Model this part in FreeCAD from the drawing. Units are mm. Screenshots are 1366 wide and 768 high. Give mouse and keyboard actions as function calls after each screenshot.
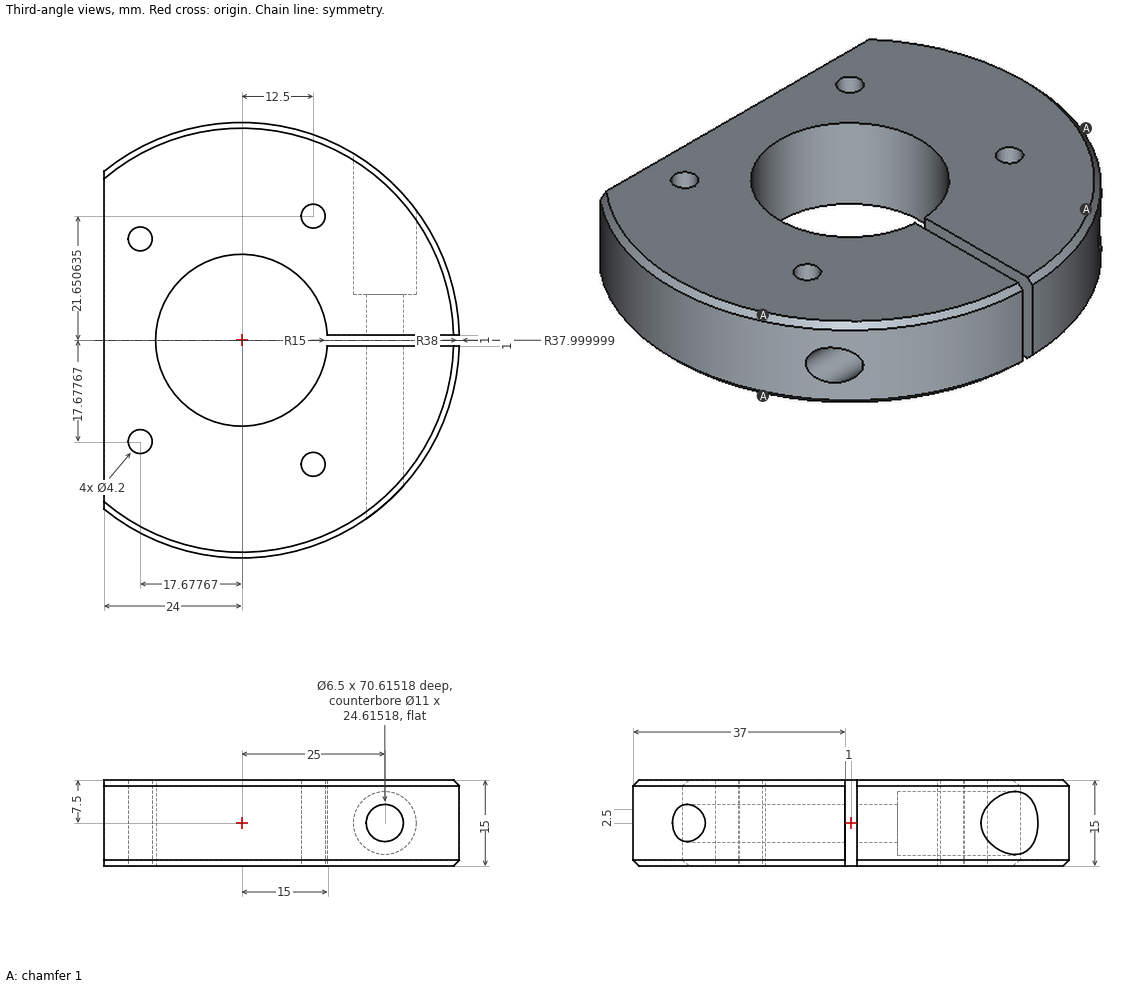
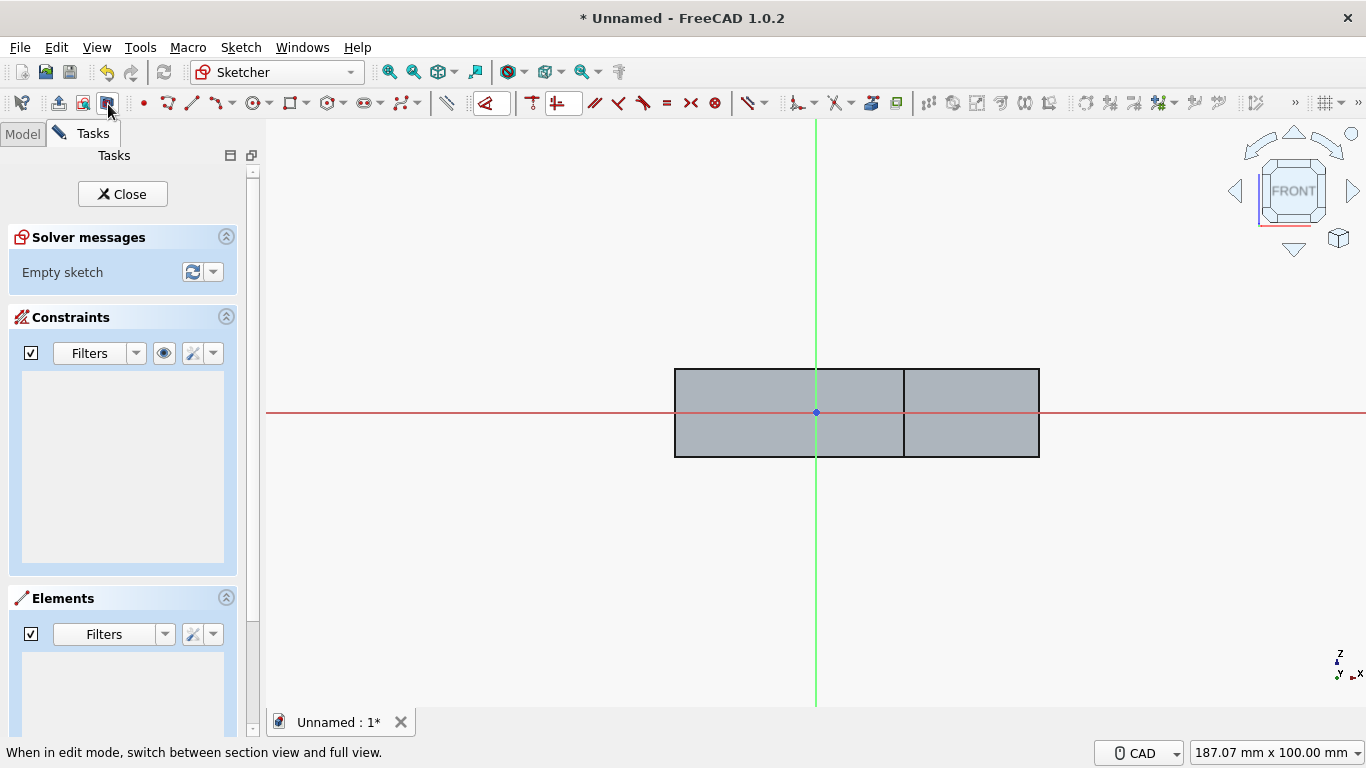
scroll(897, 413, up, 7)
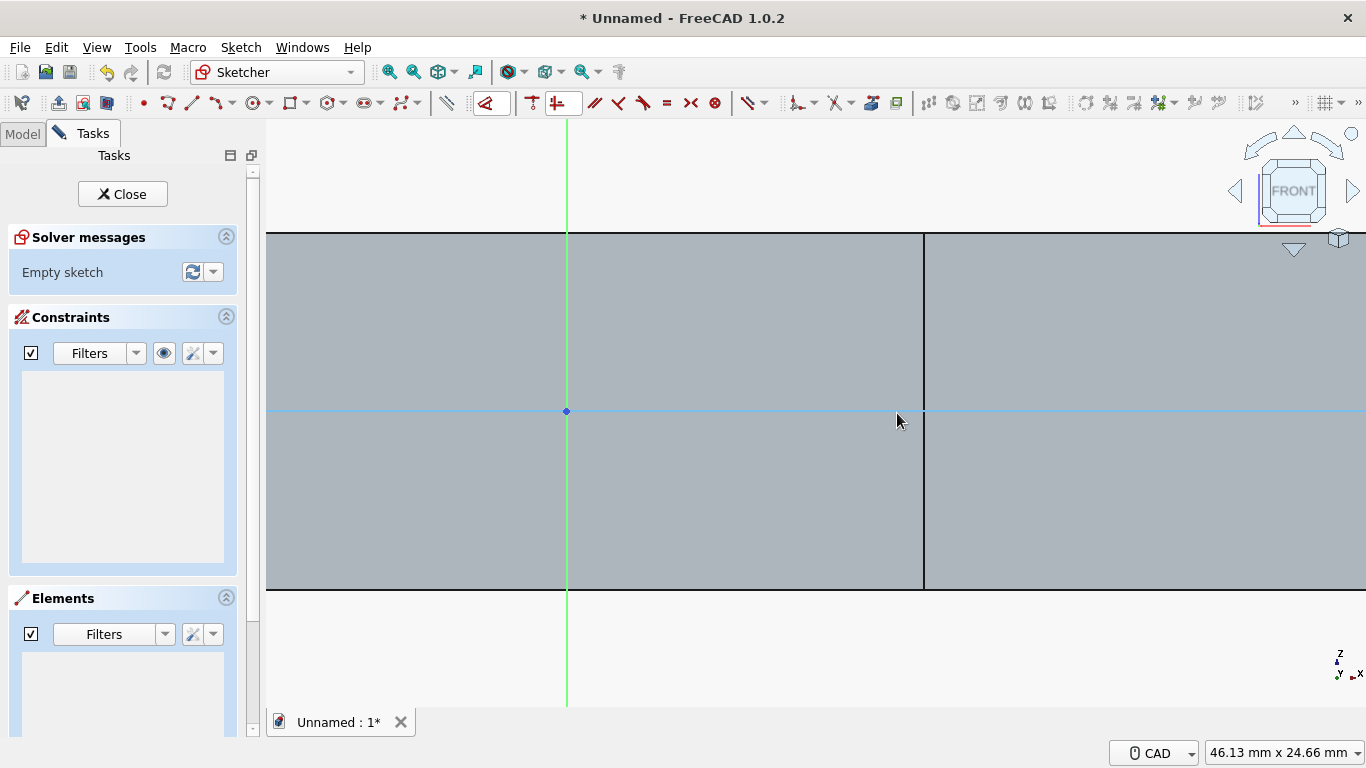
key(g)
key(r)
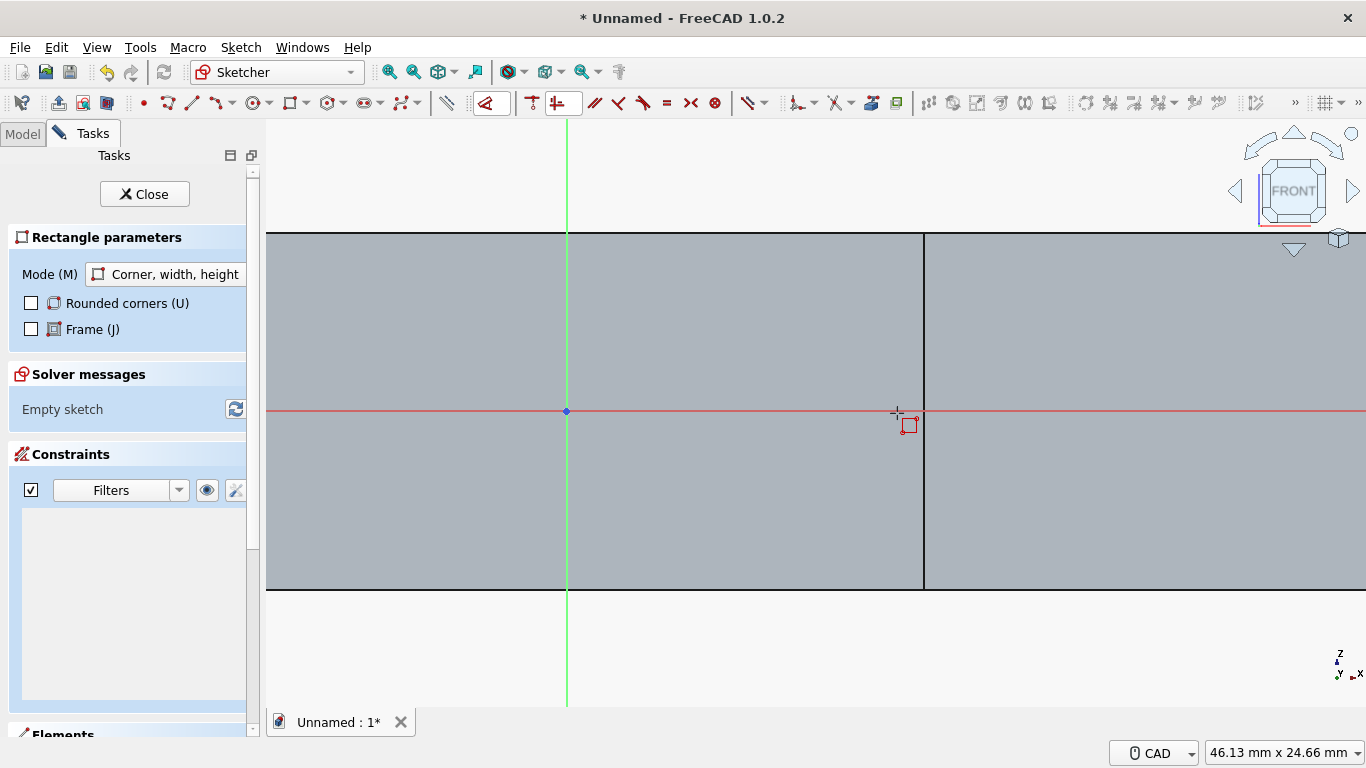
click(567, 233)
move(924, 590)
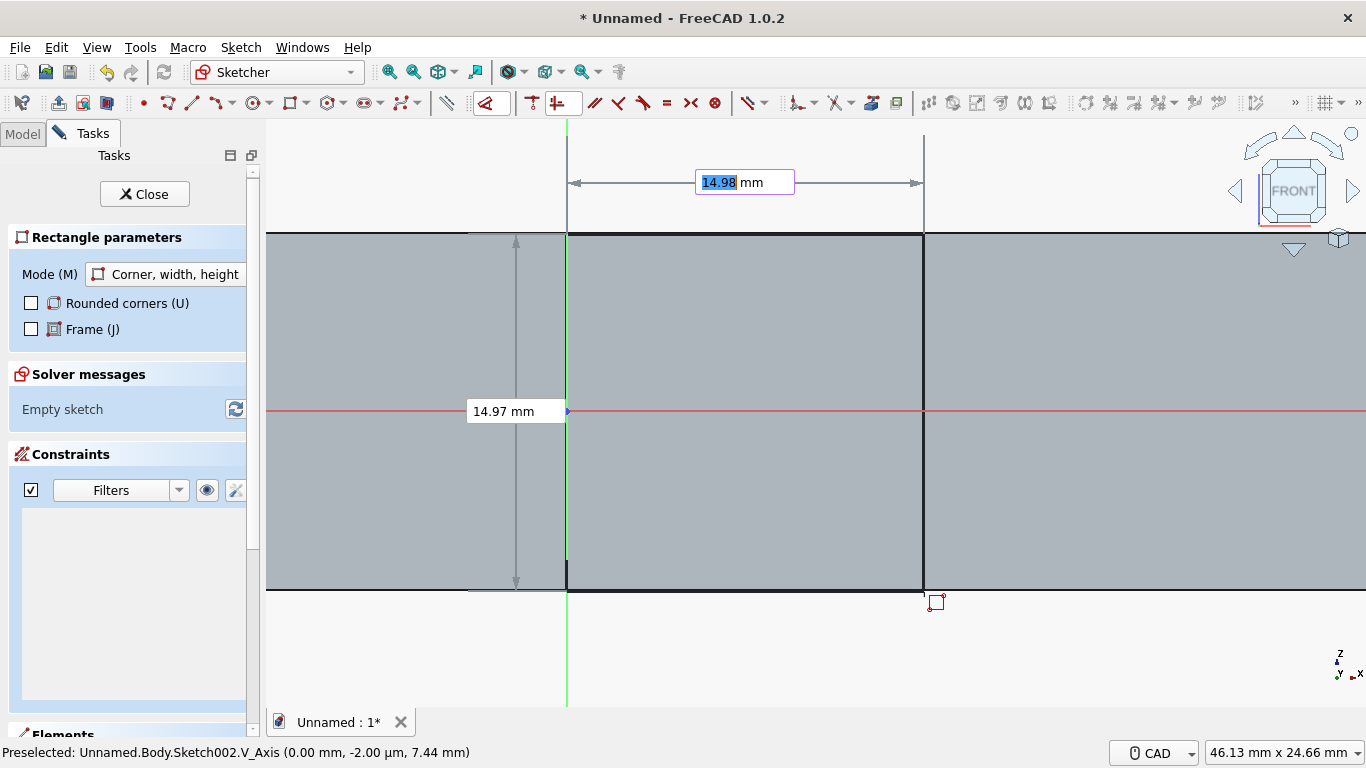
text(15)
key(Tab)
text(15)
key(Return)
key(Escape)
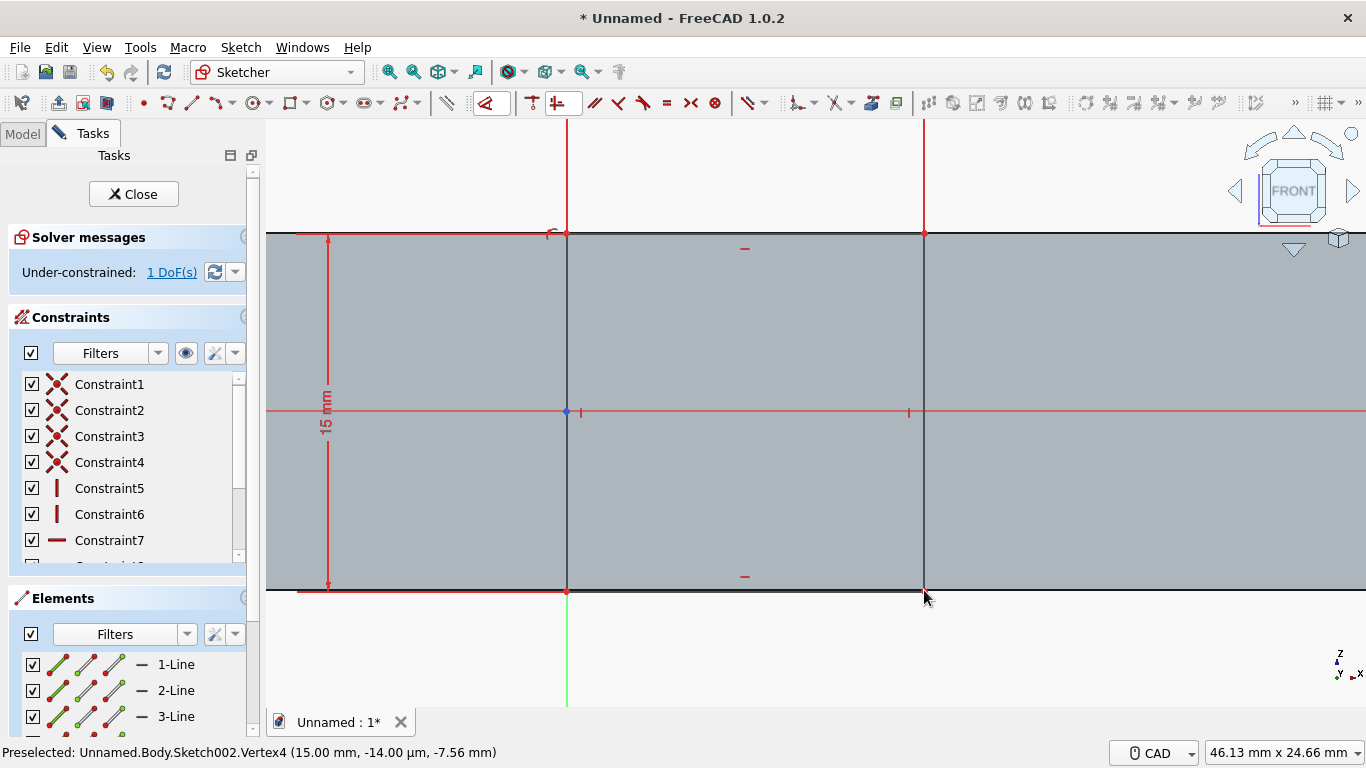
click(567, 234)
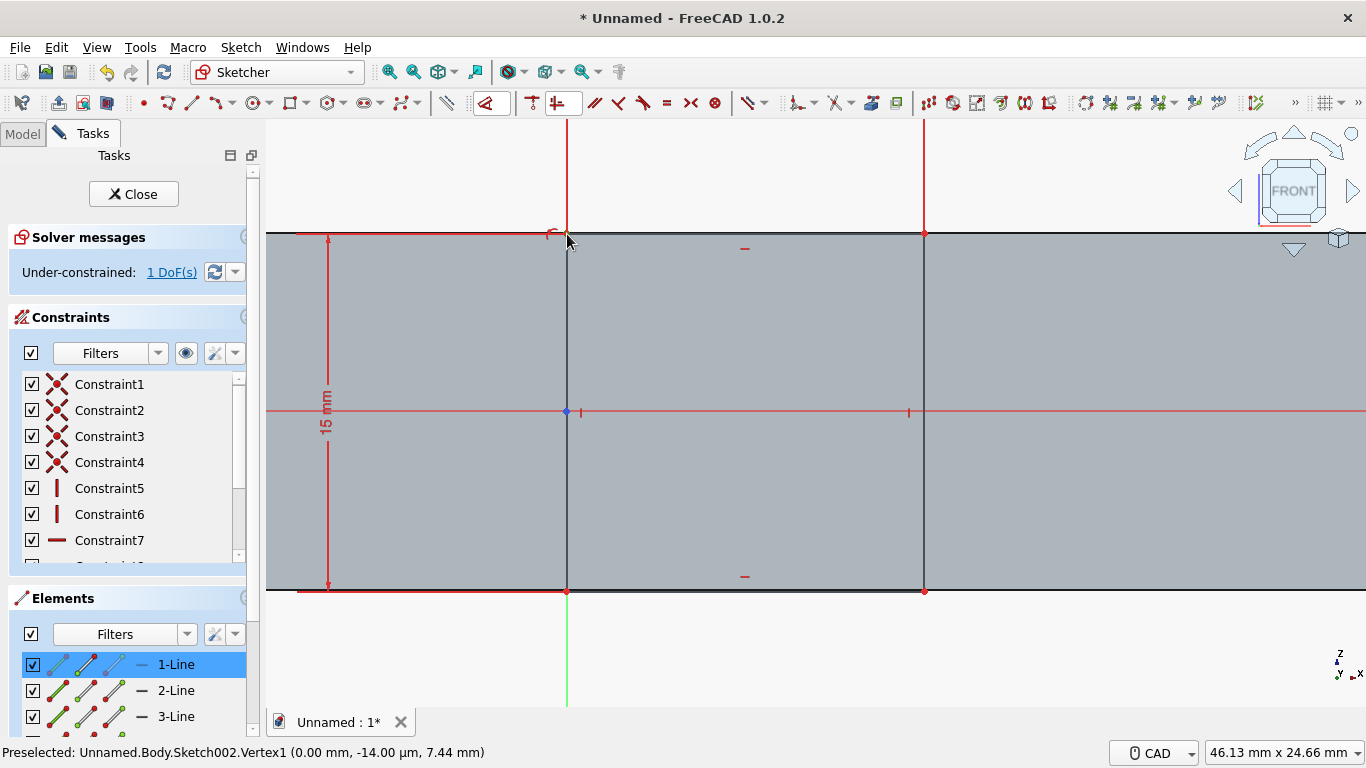
click(504, 104)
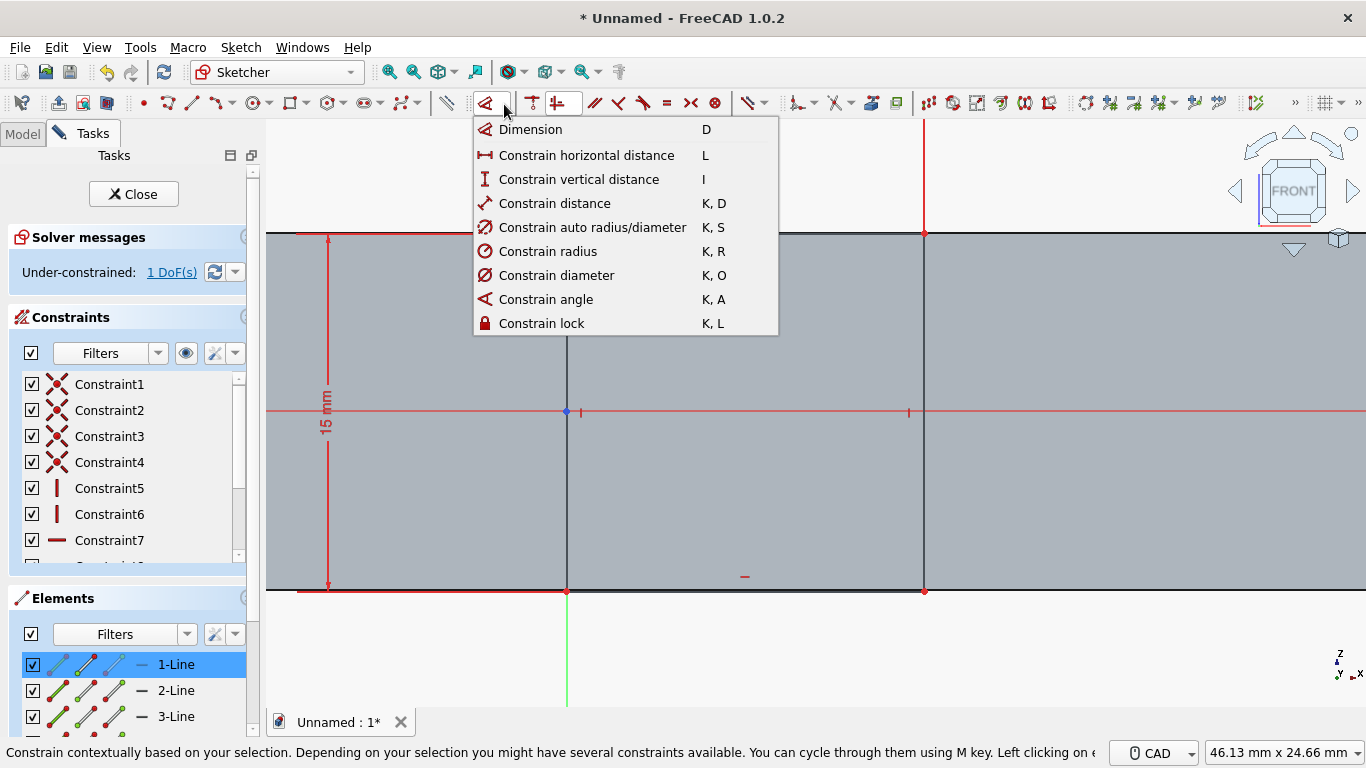
click(626, 179)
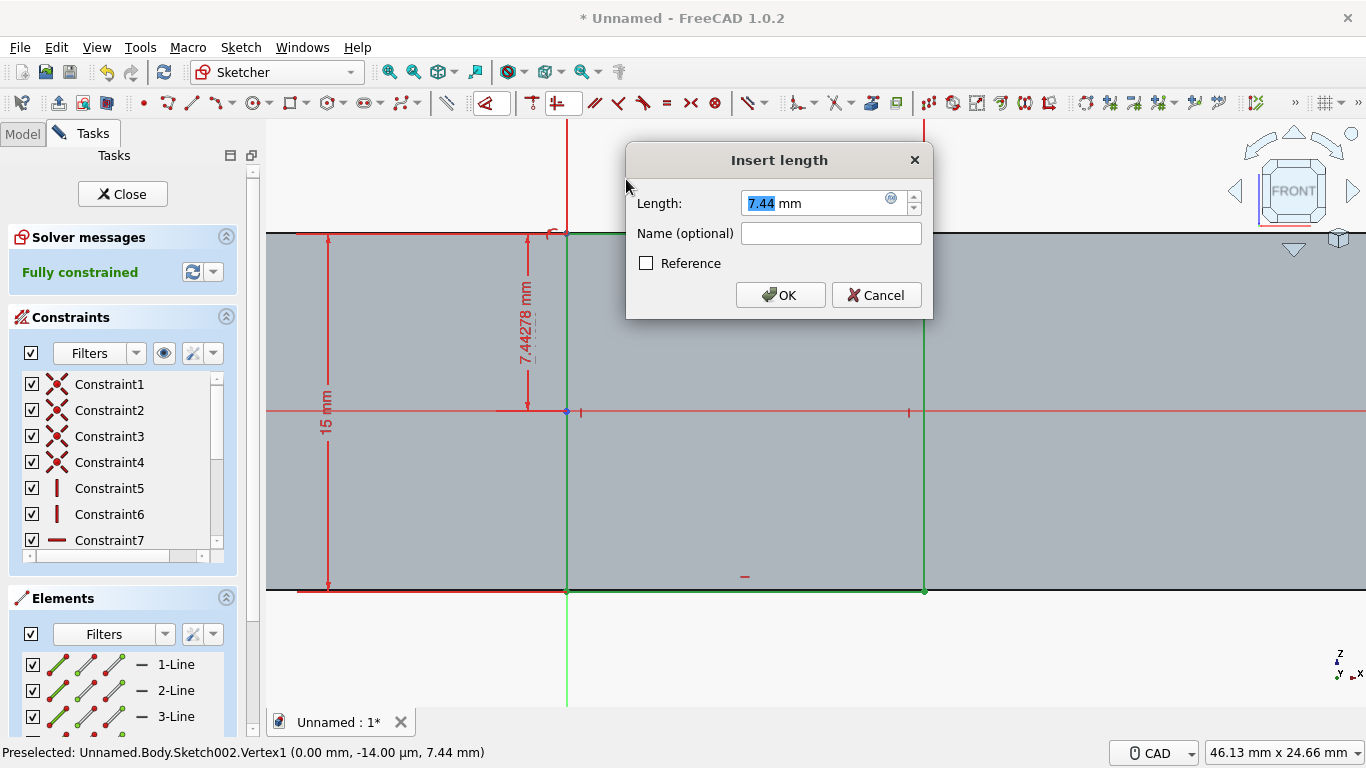
text(7.5)
key(Return)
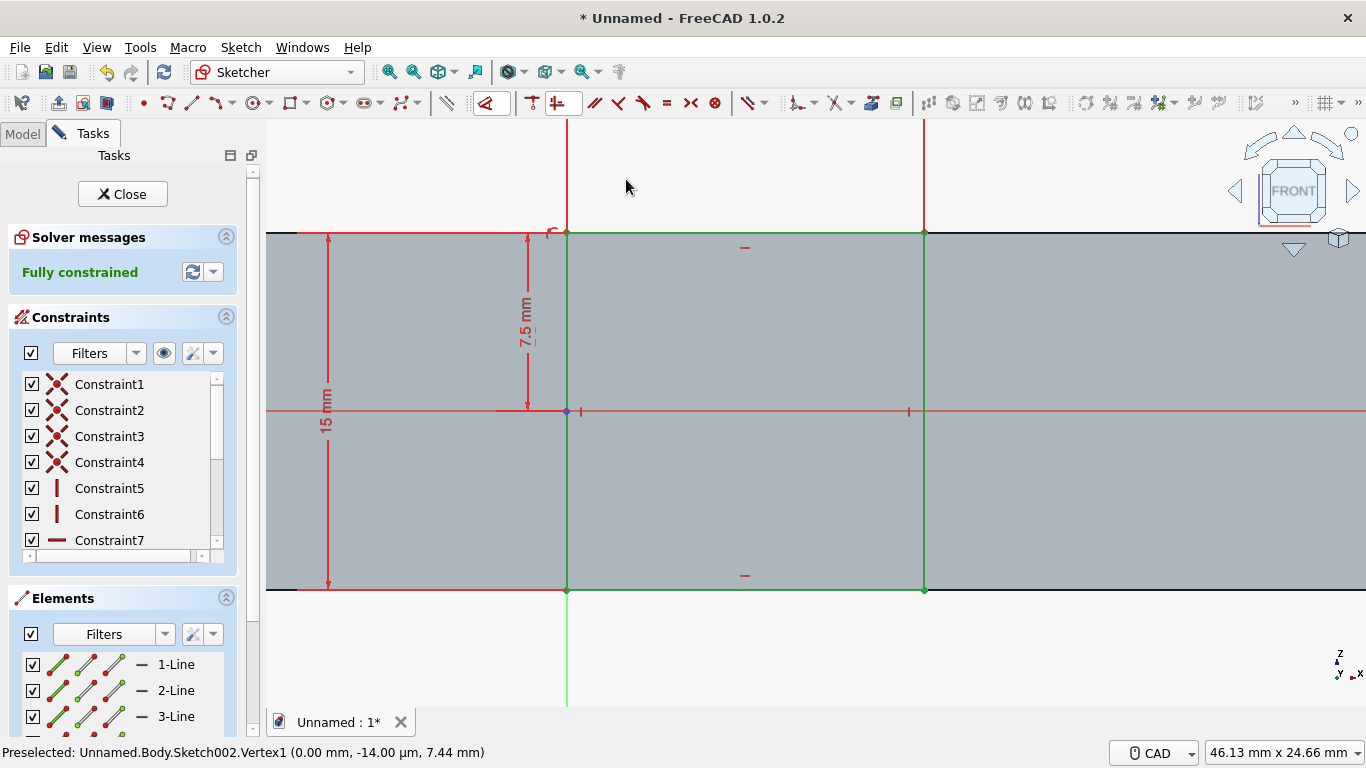
click(123, 194)